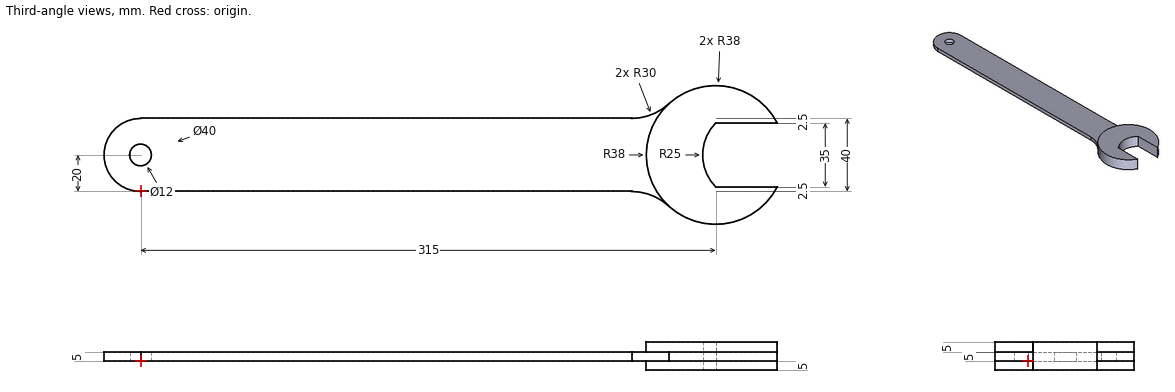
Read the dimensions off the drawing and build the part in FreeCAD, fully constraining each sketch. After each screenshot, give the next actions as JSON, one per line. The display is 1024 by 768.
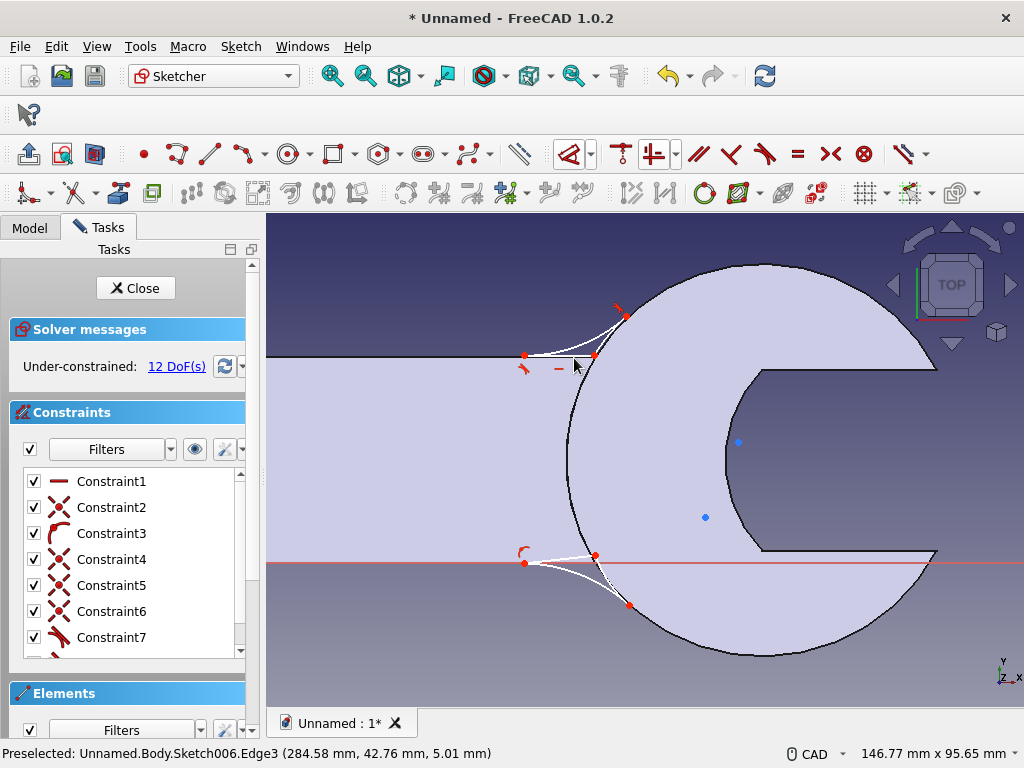
{"action": "scroll", "coordinate": [574, 558], "scroll_direction": "up", "scroll_amount": 5}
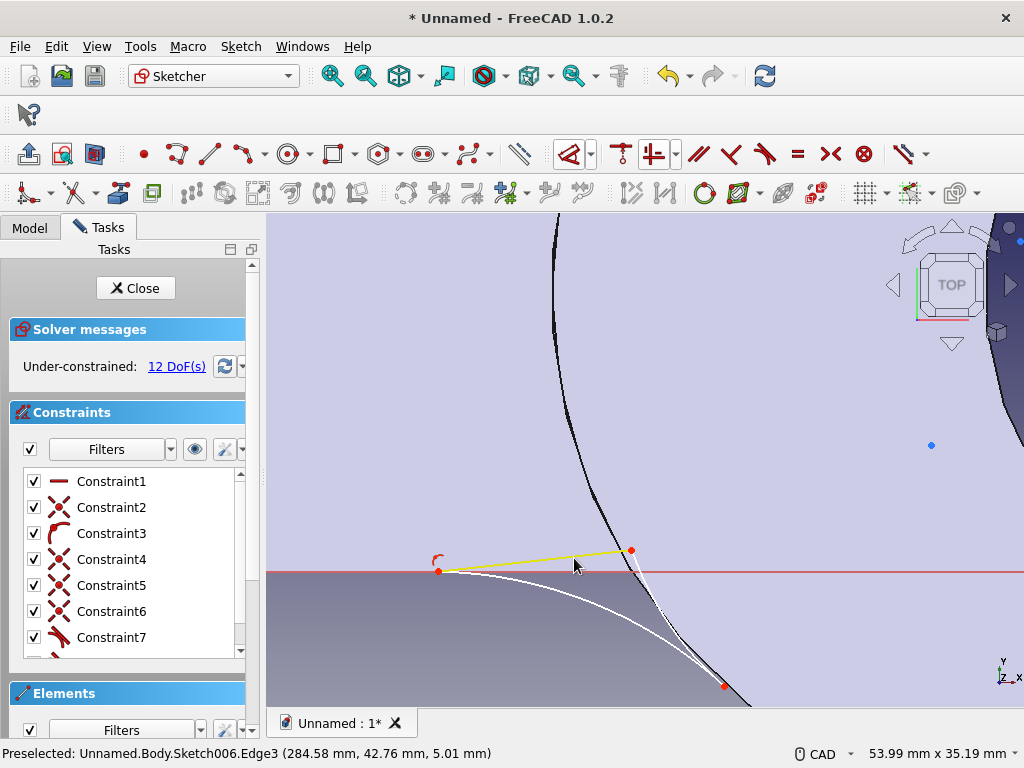
{"action": "left_click", "coordinate": [574, 557]}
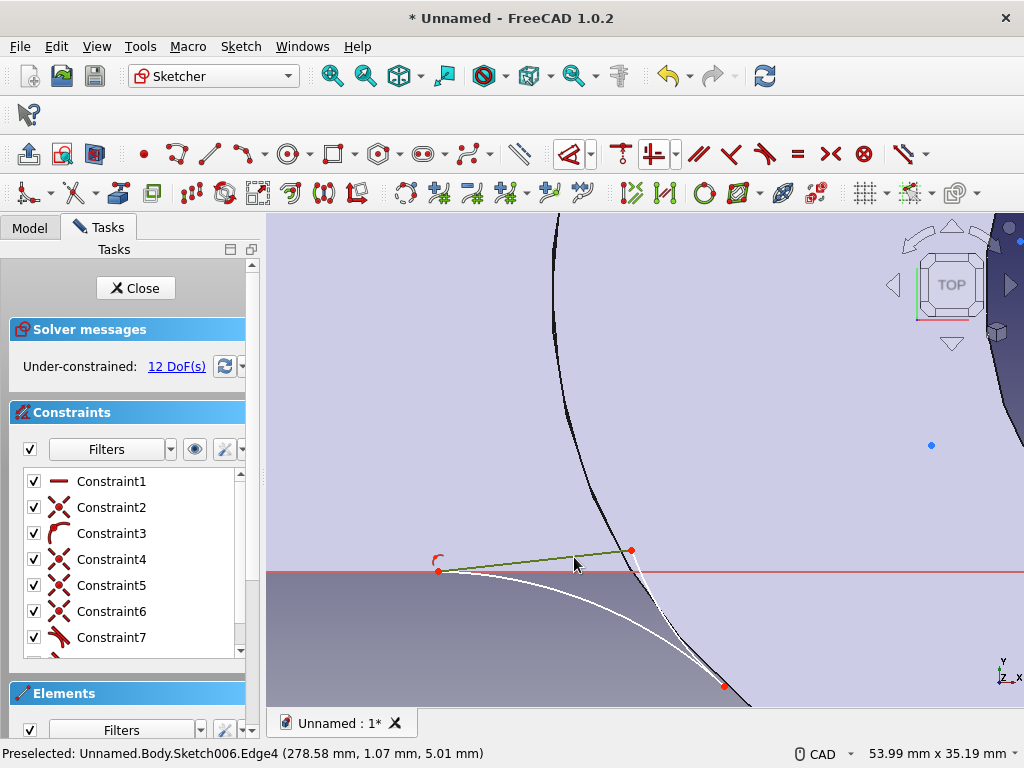
{"action": "left_click", "coordinate": [648, 630]}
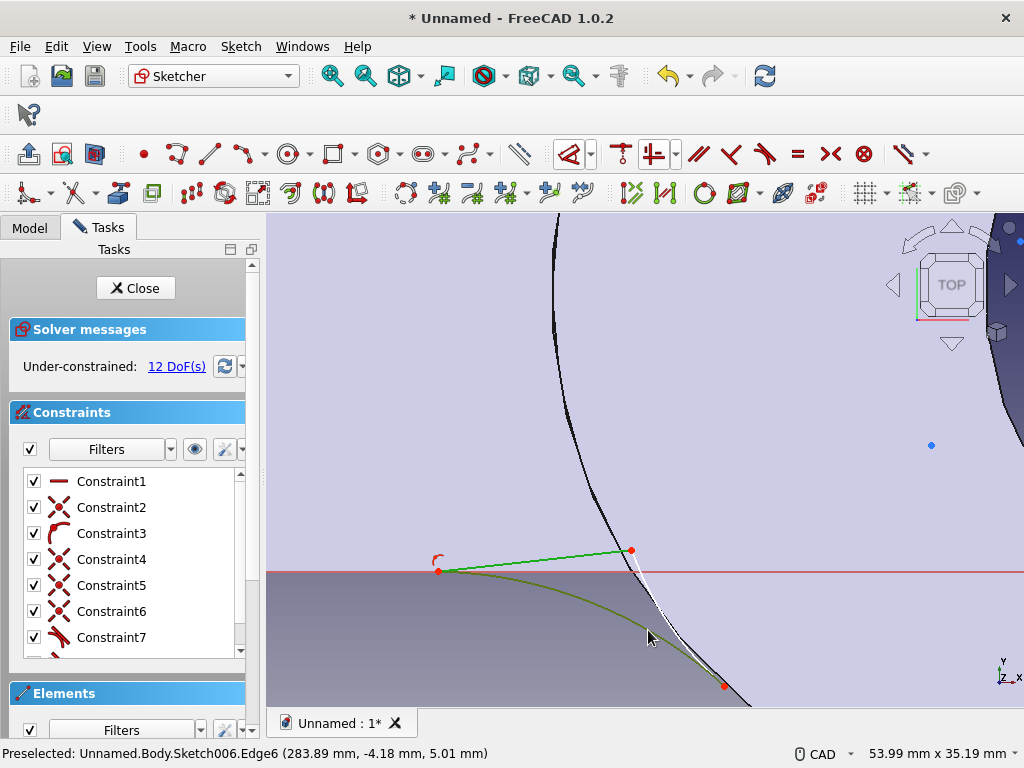
{"action": "left_click", "coordinate": [765, 154]}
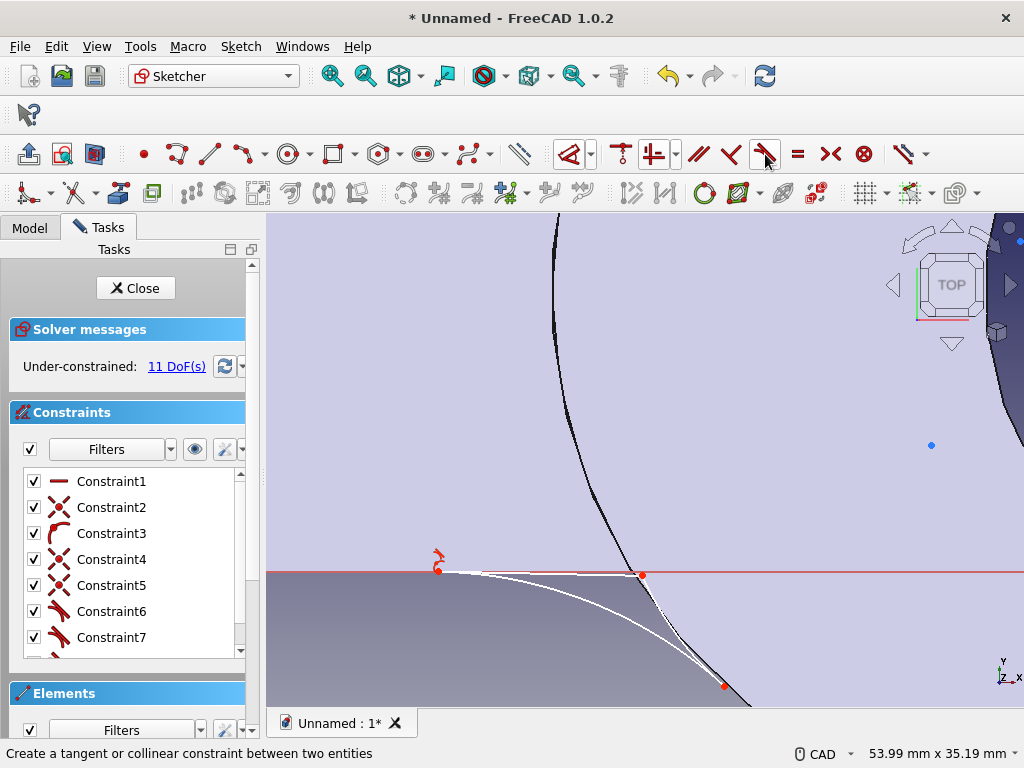
{"action": "left_click", "coordinate": [662, 613]}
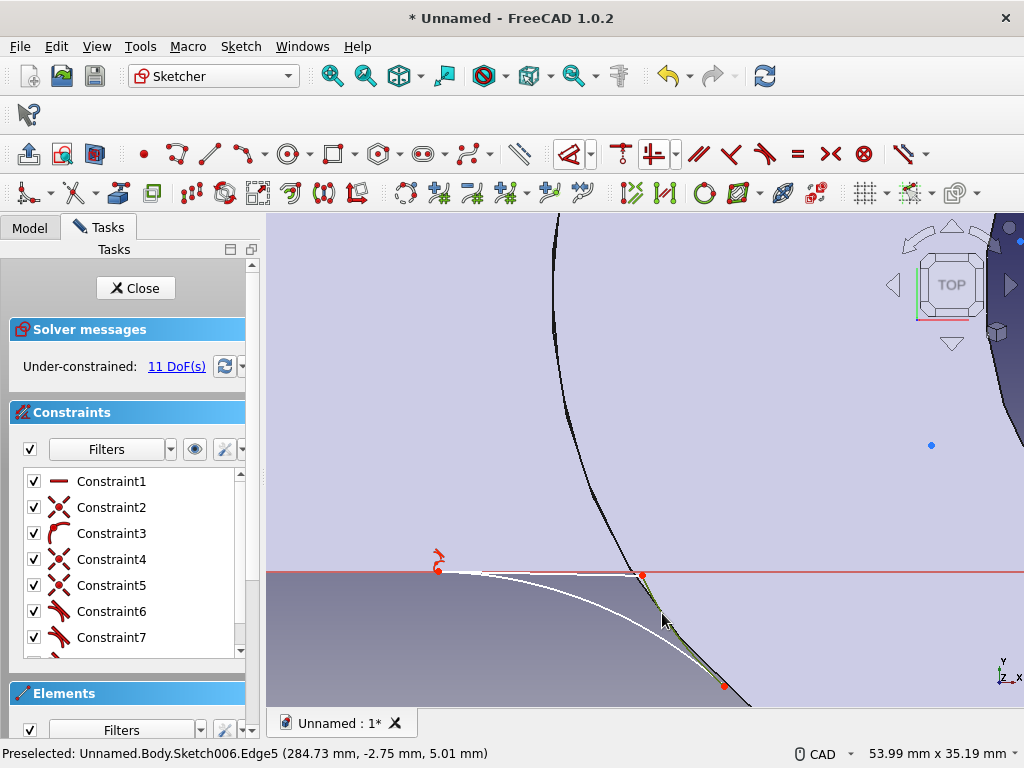
{"action": "left_click", "coordinate": [648, 630]}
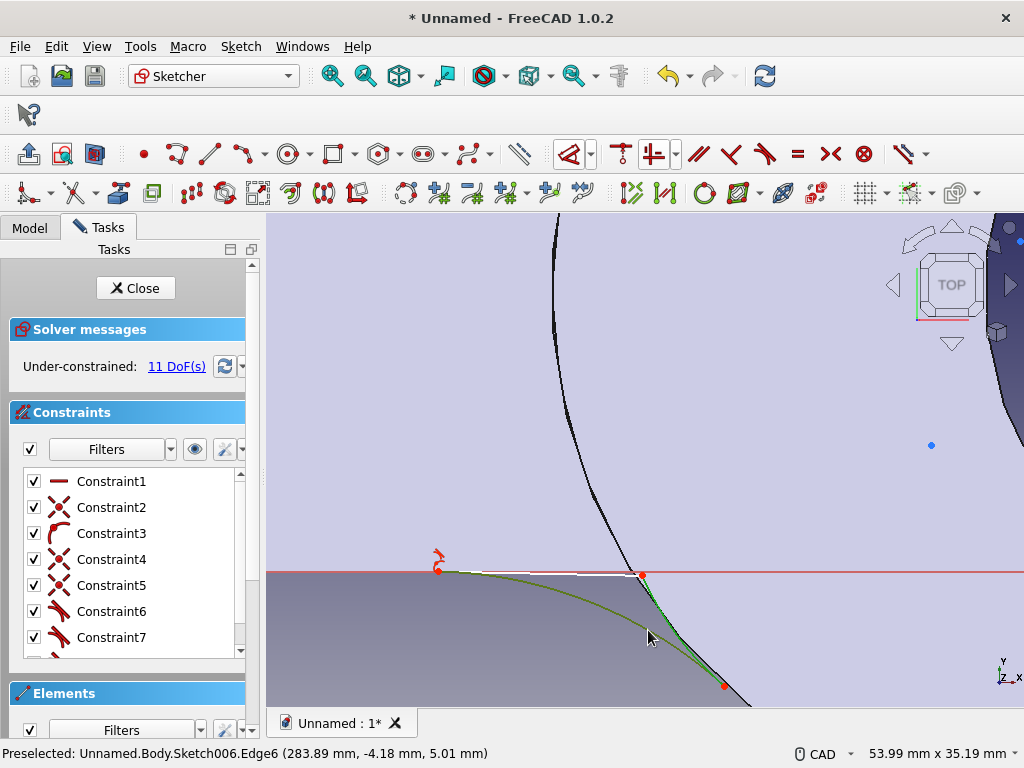
{"action": "left_click", "coordinate": [765, 154]}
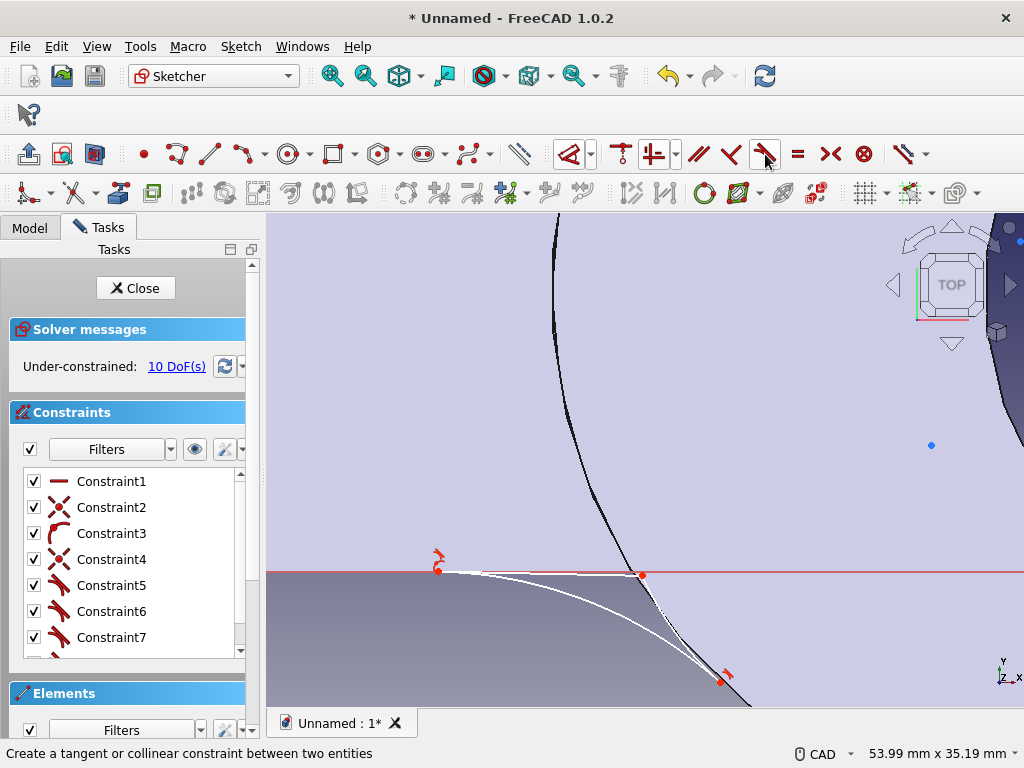
{"action": "left_click", "coordinate": [581, 575]}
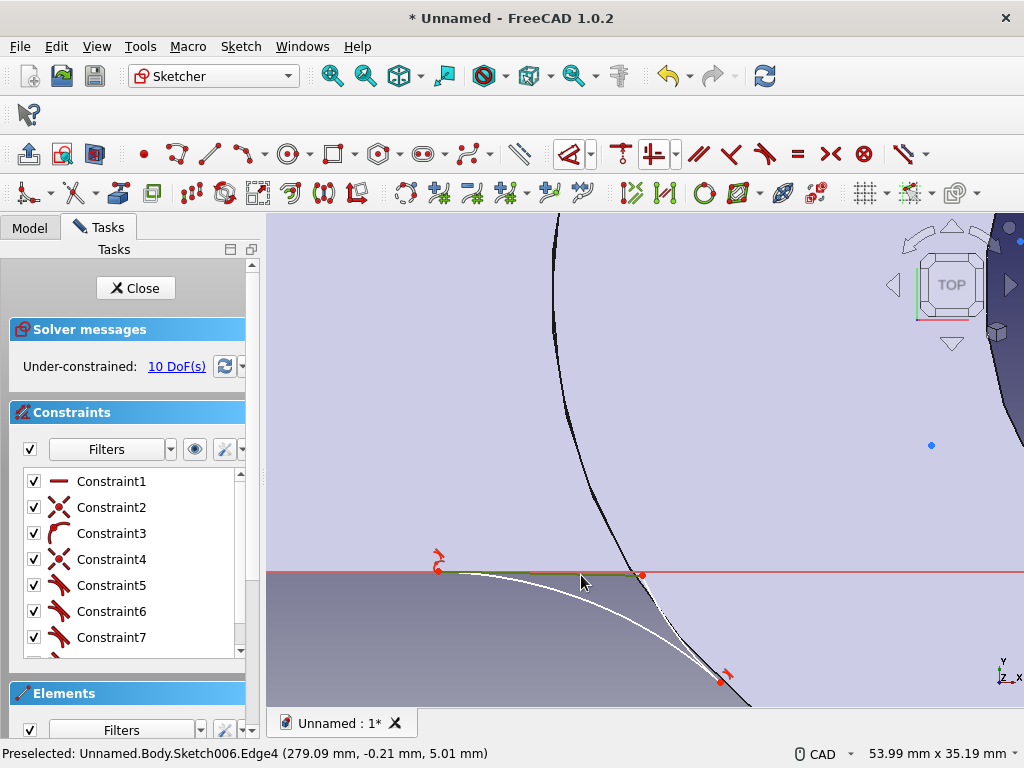
{"action": "left_click", "coordinate": [676, 154]}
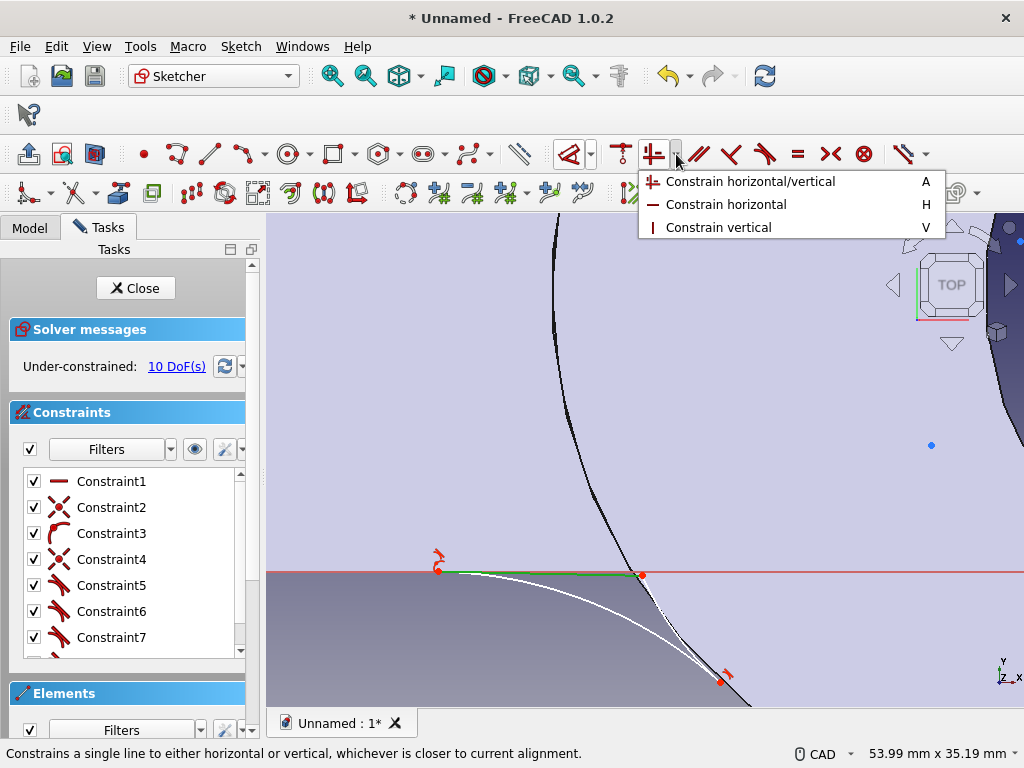
{"action": "left_click", "coordinate": [792, 204]}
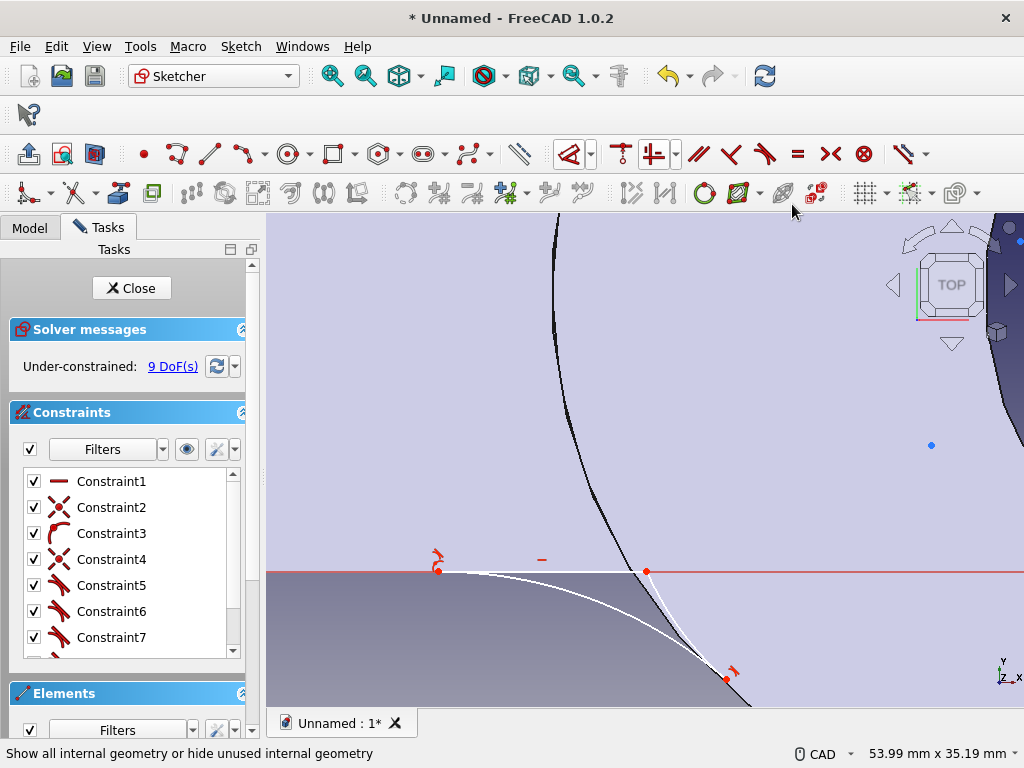
{"action": "scroll", "coordinate": [574, 558], "scroll_direction": "down", "scroll_amount": 5}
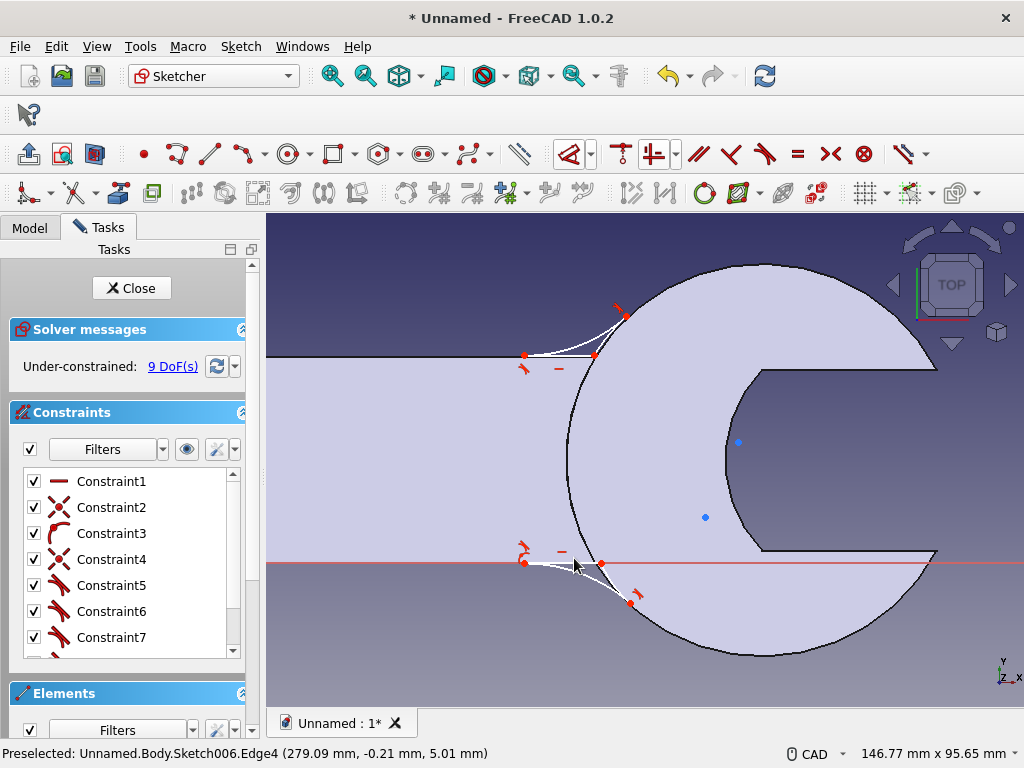
{"action": "scroll", "coordinate": [603, 343], "scroll_direction": "up", "scroll_amount": 3}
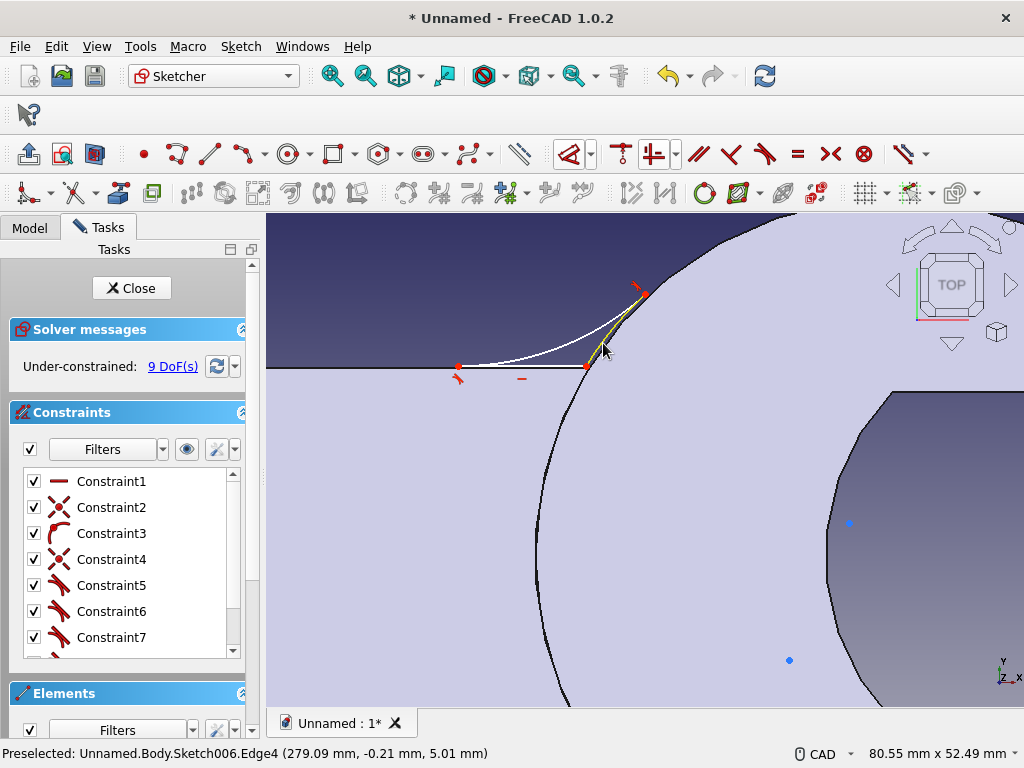
{"action": "left_click", "coordinate": [602, 343]}